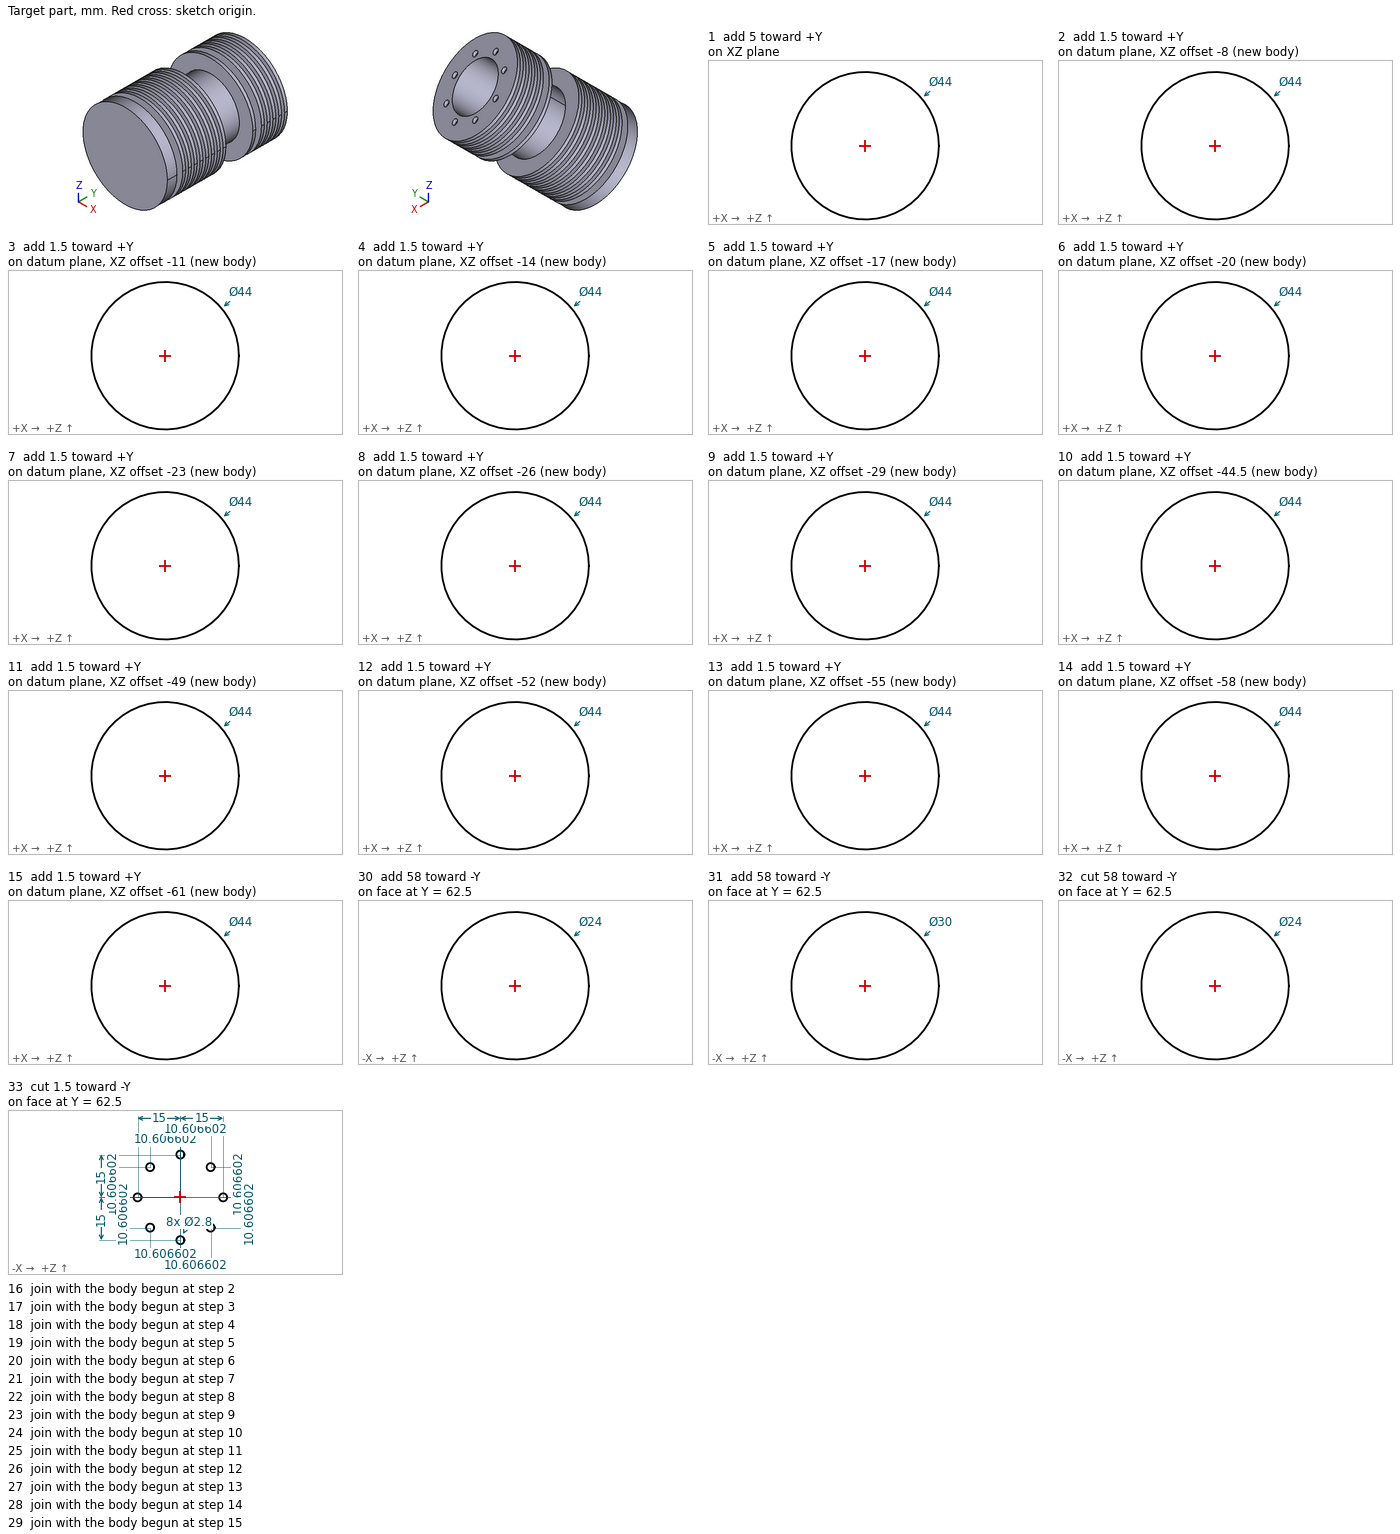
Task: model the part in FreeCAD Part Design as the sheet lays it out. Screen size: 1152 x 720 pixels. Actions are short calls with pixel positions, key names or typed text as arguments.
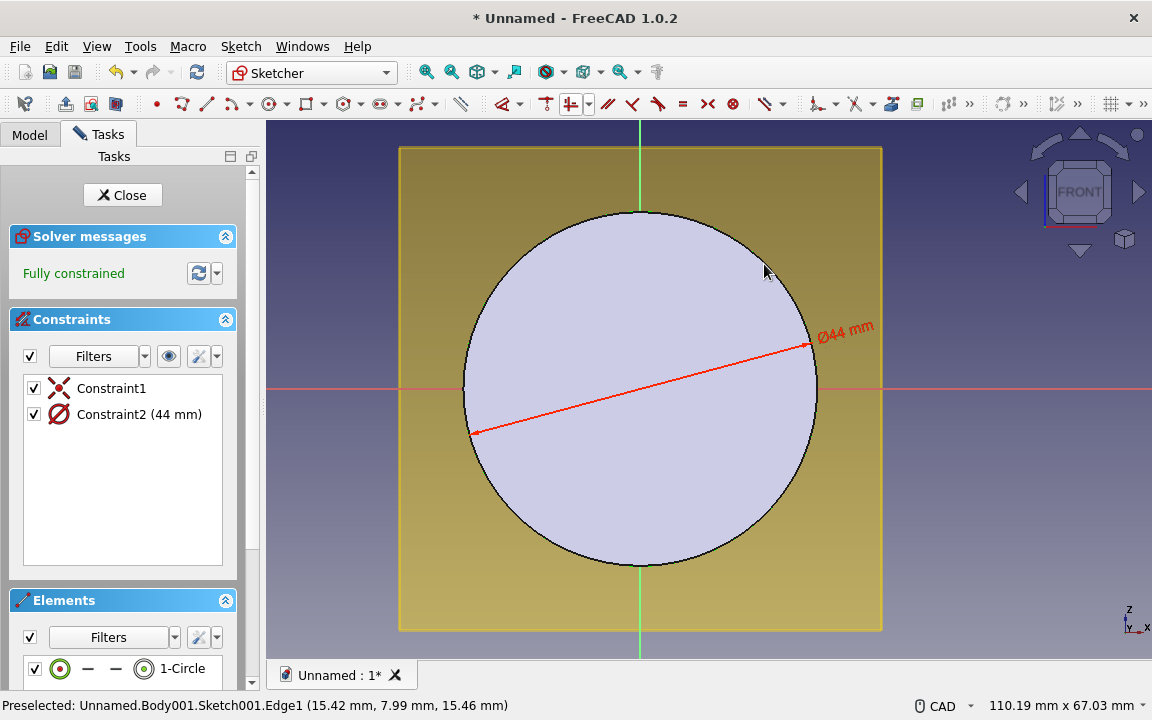
click(123, 195)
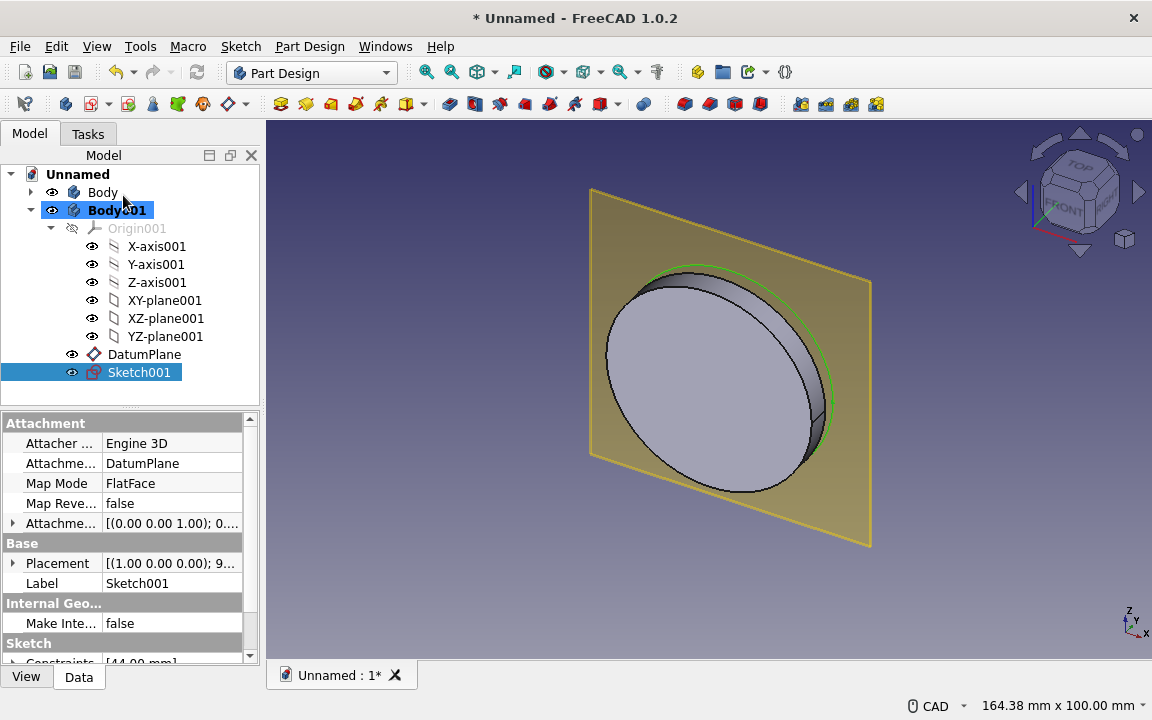
click(281, 104)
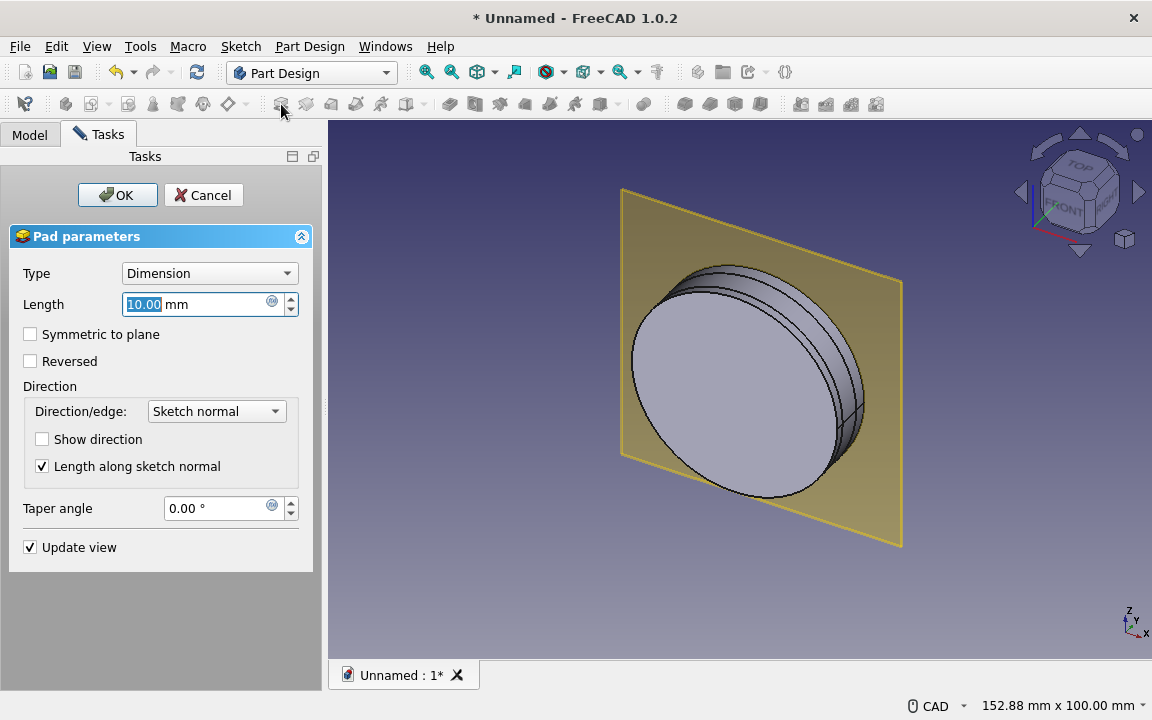
text(1.5)
key(Tab)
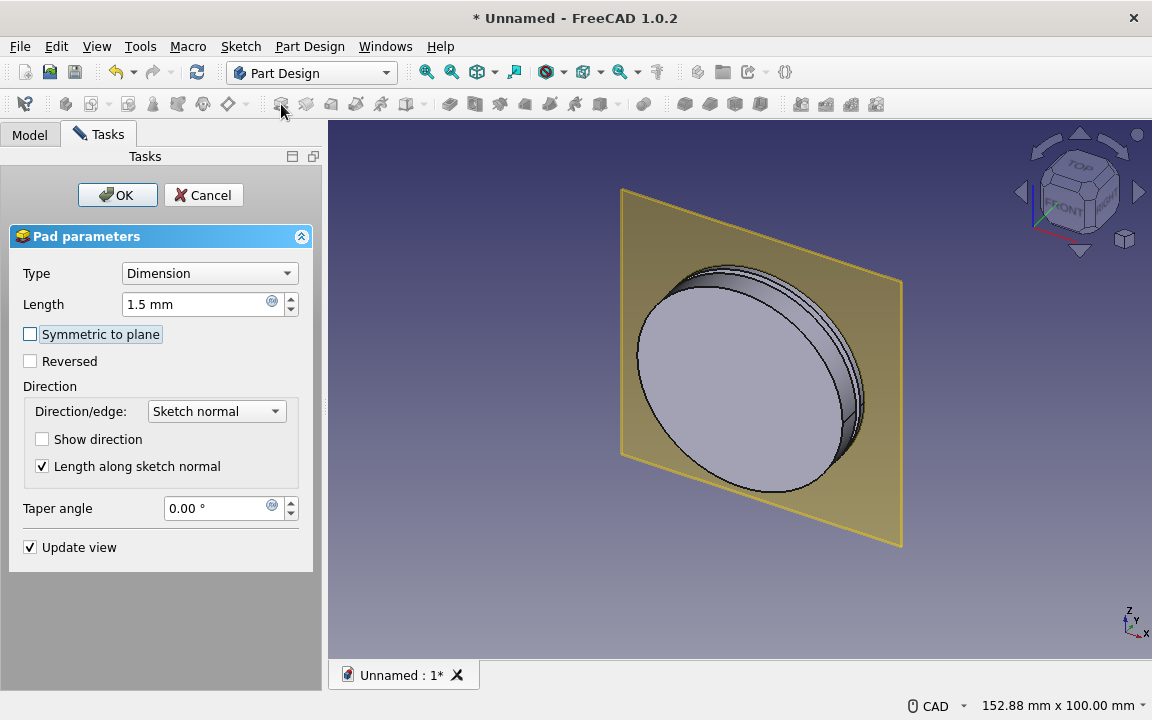
click(31, 361)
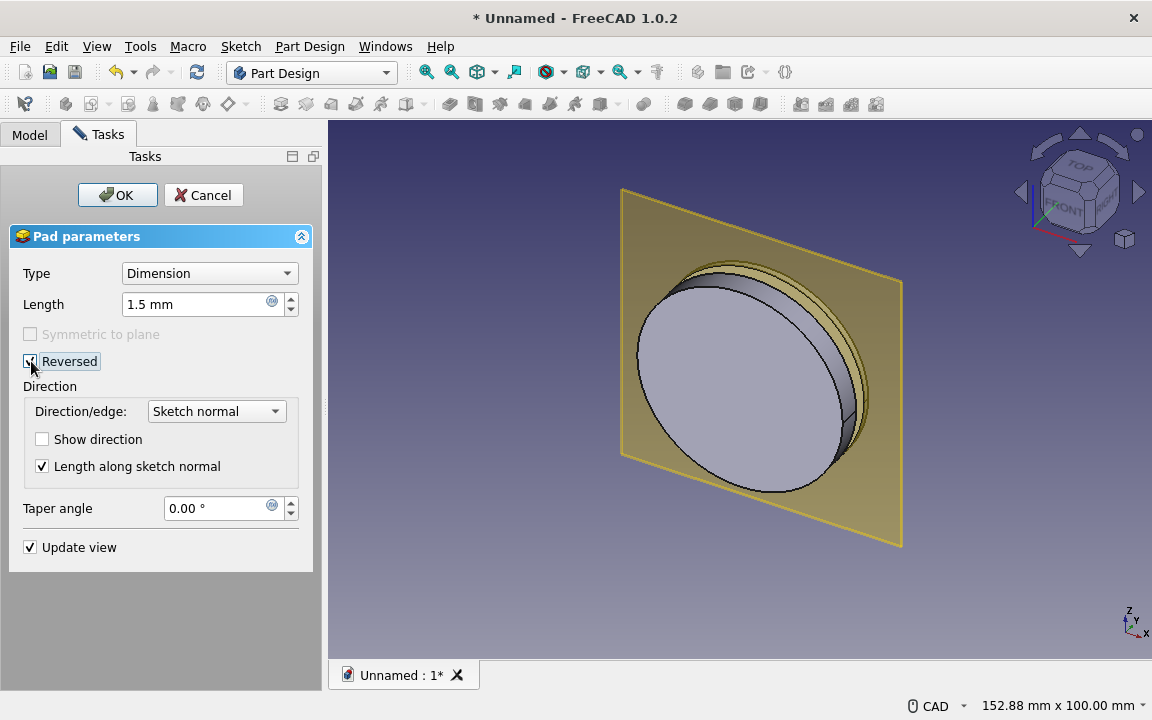
click(118, 195)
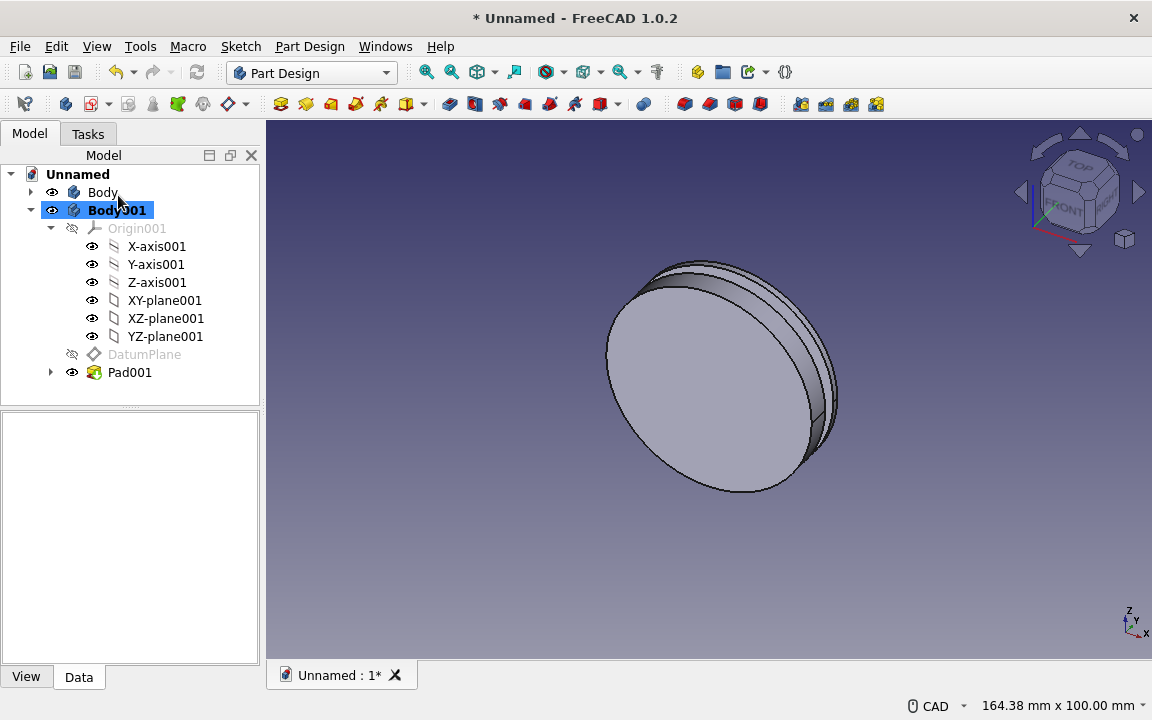
click(66, 104)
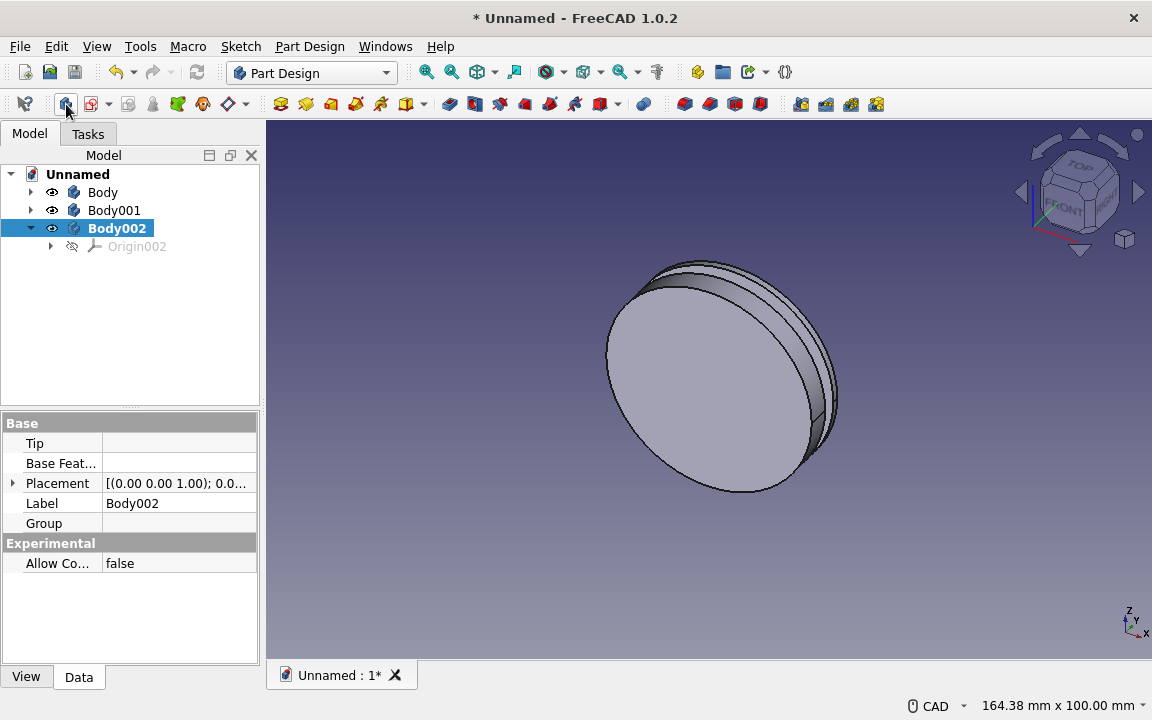
click(51, 246)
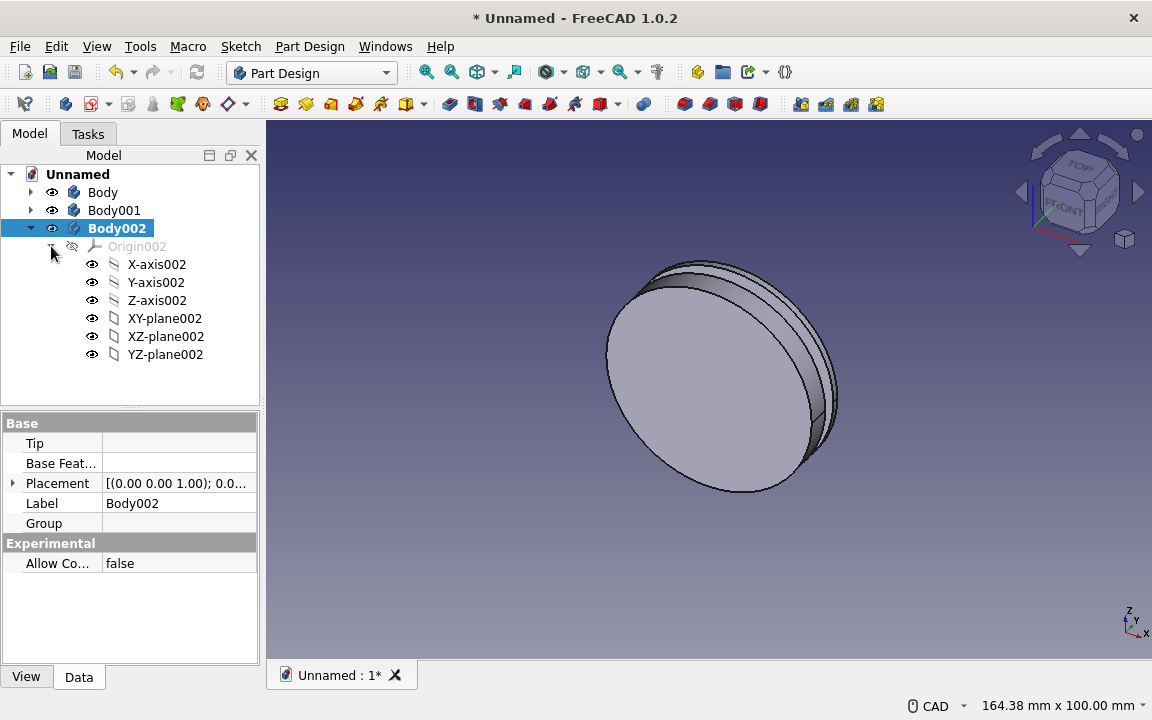
click(137, 336)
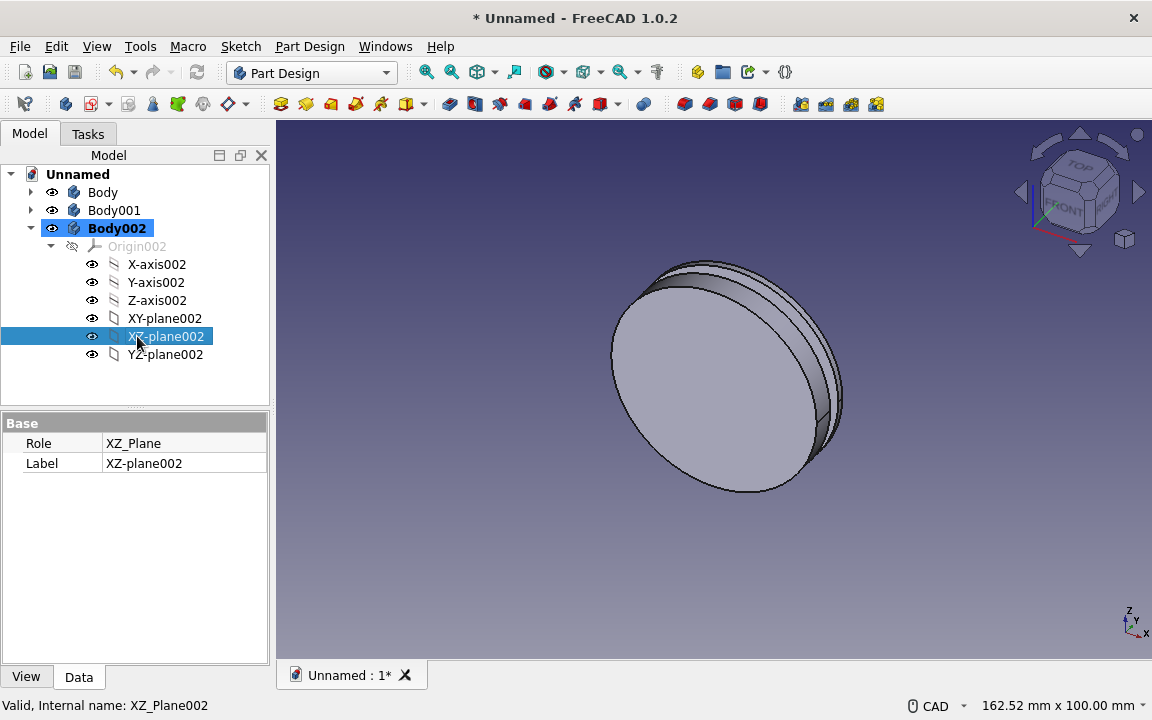
click(228, 104)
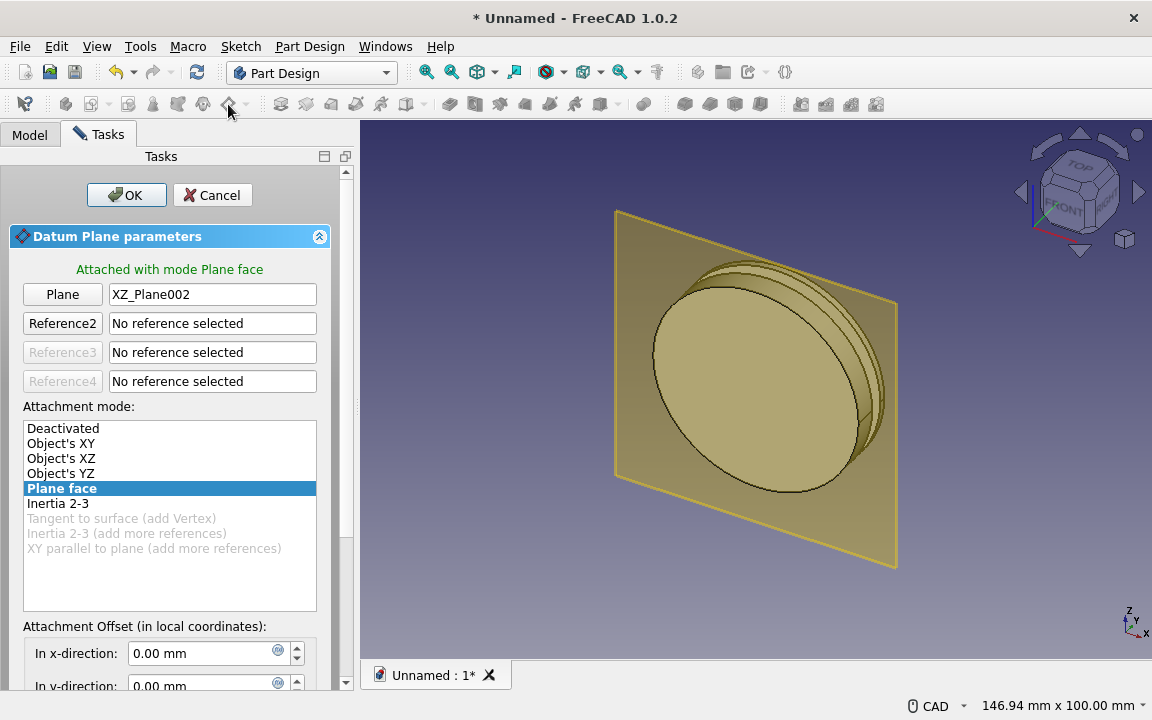
scroll(346, 428, down, 2)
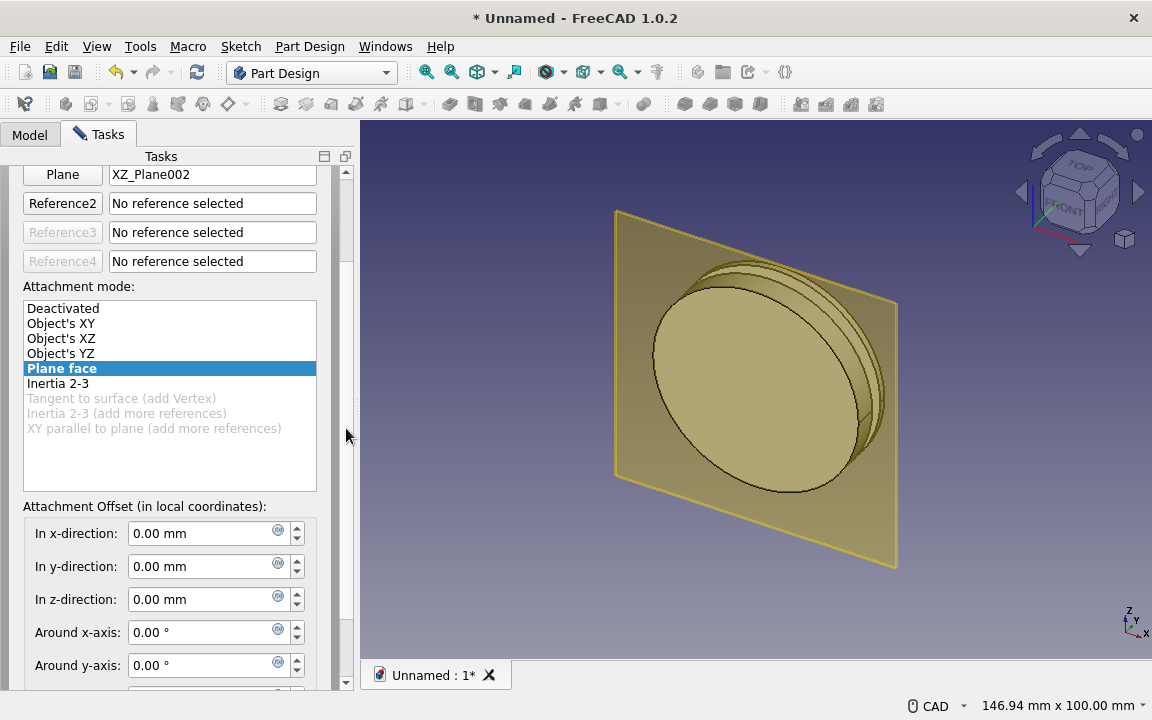
triple_click(210, 600)